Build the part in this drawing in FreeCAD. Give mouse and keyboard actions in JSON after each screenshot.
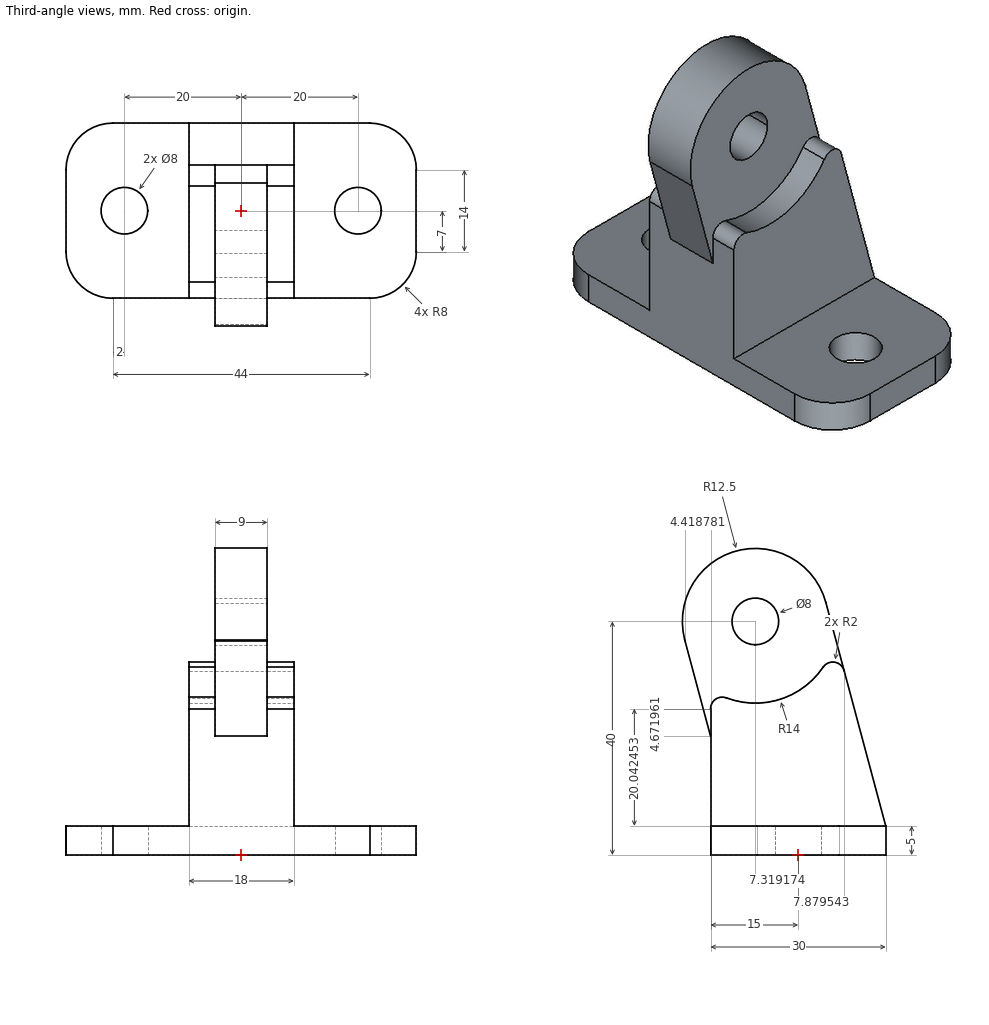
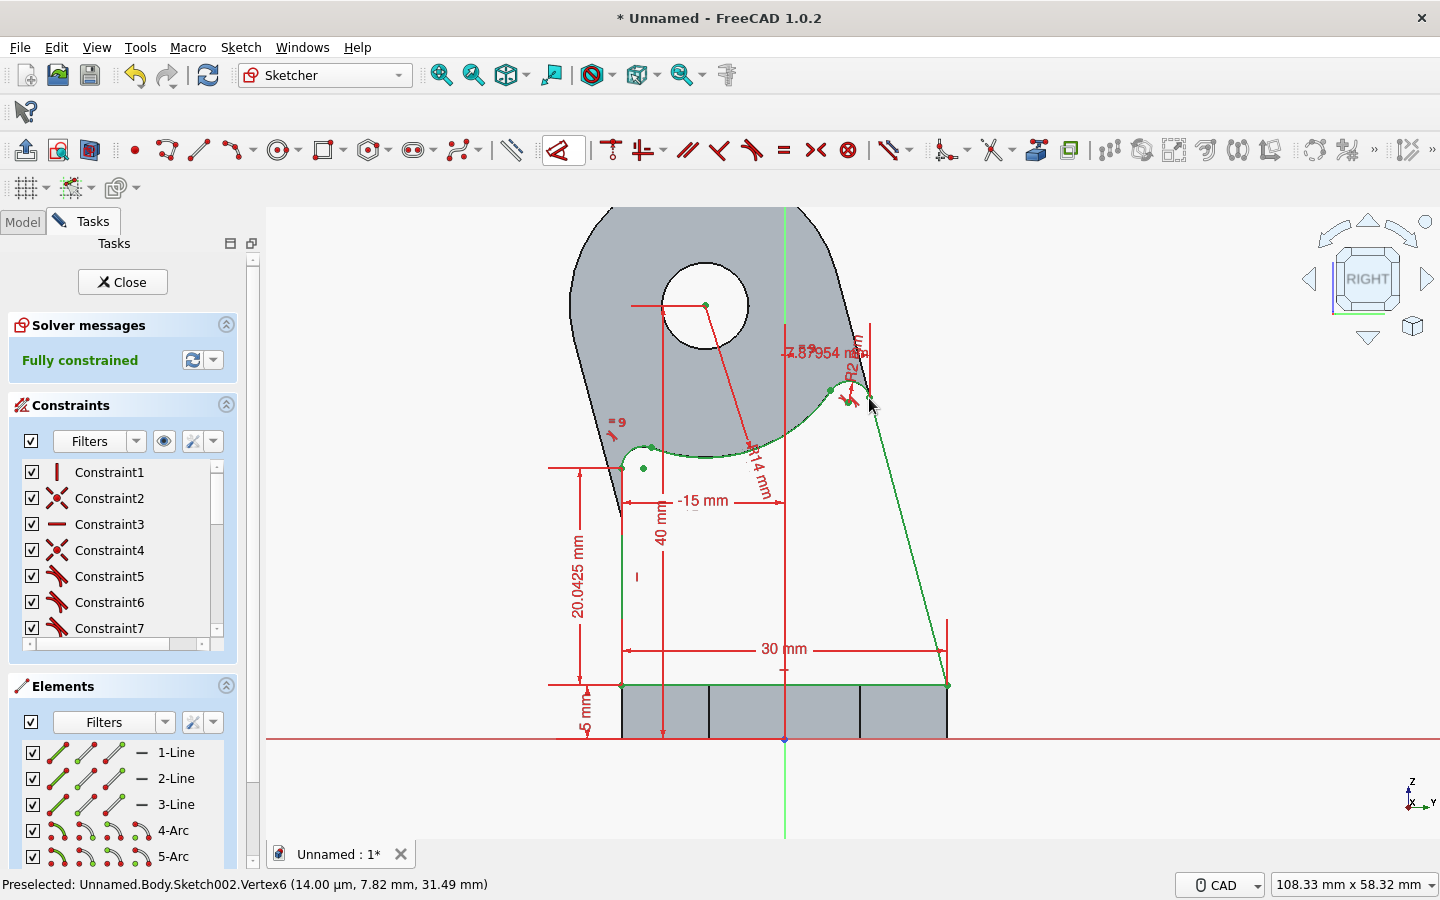
{"action": "left_click", "coordinate": [123, 282]}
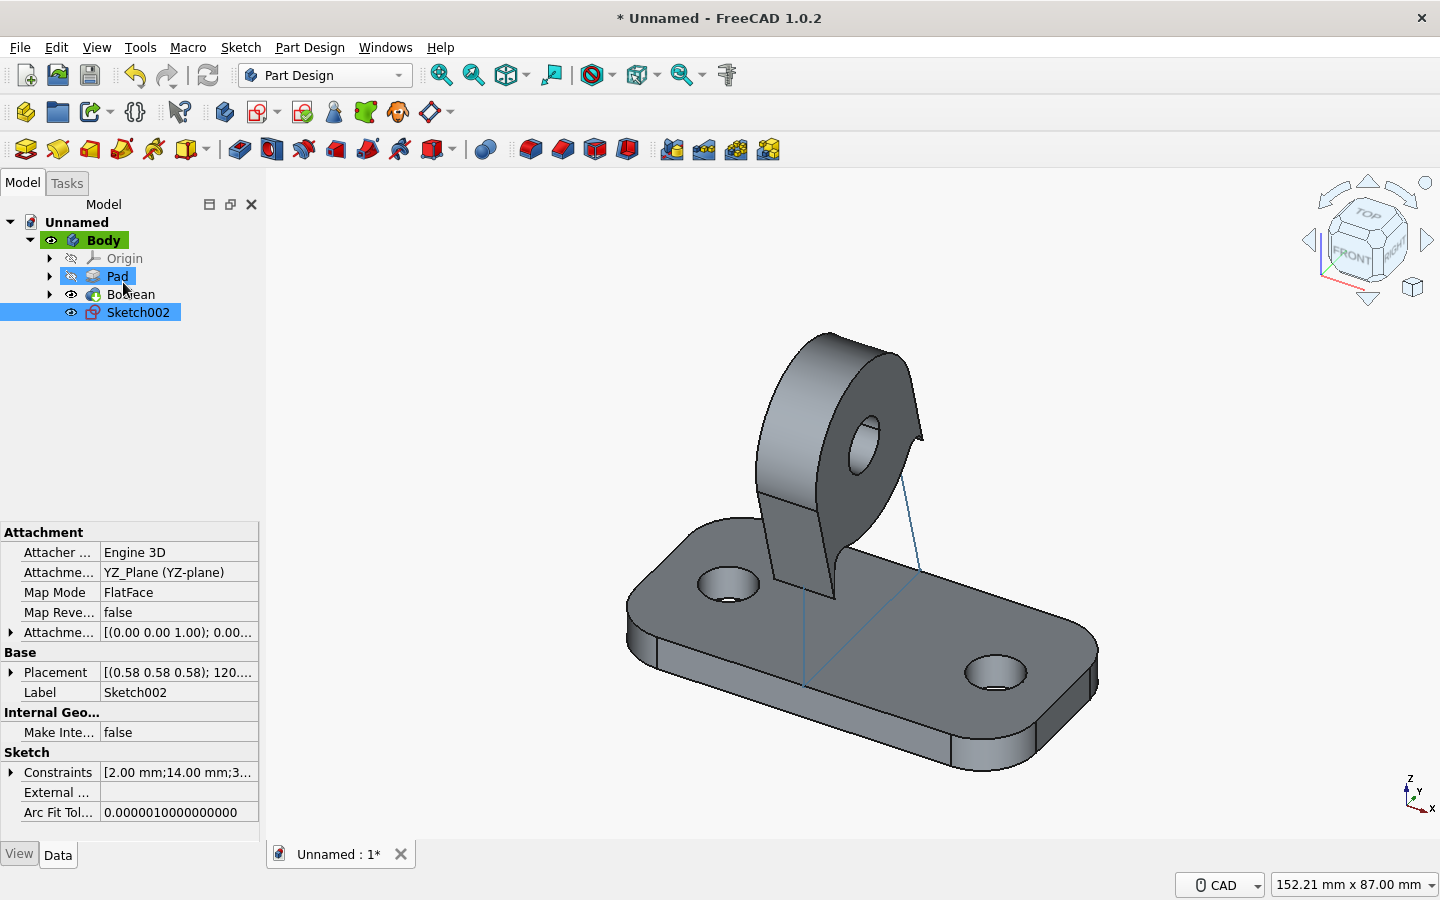
{"action": "left_click", "coordinate": [26, 150]}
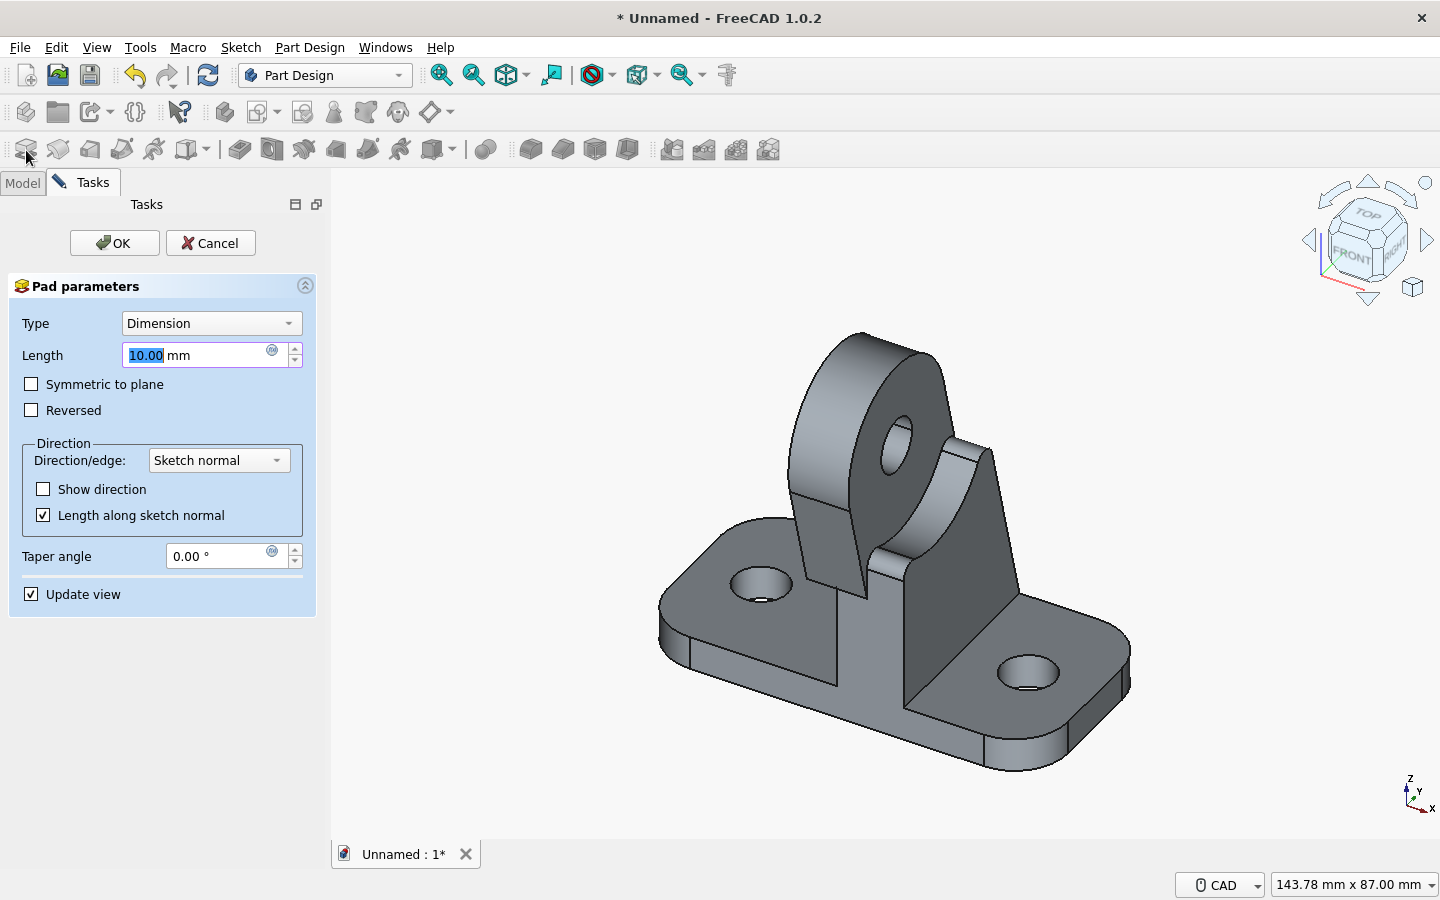
{"action": "type", "text": "18"}
{"action": "key", "text": "Tab"}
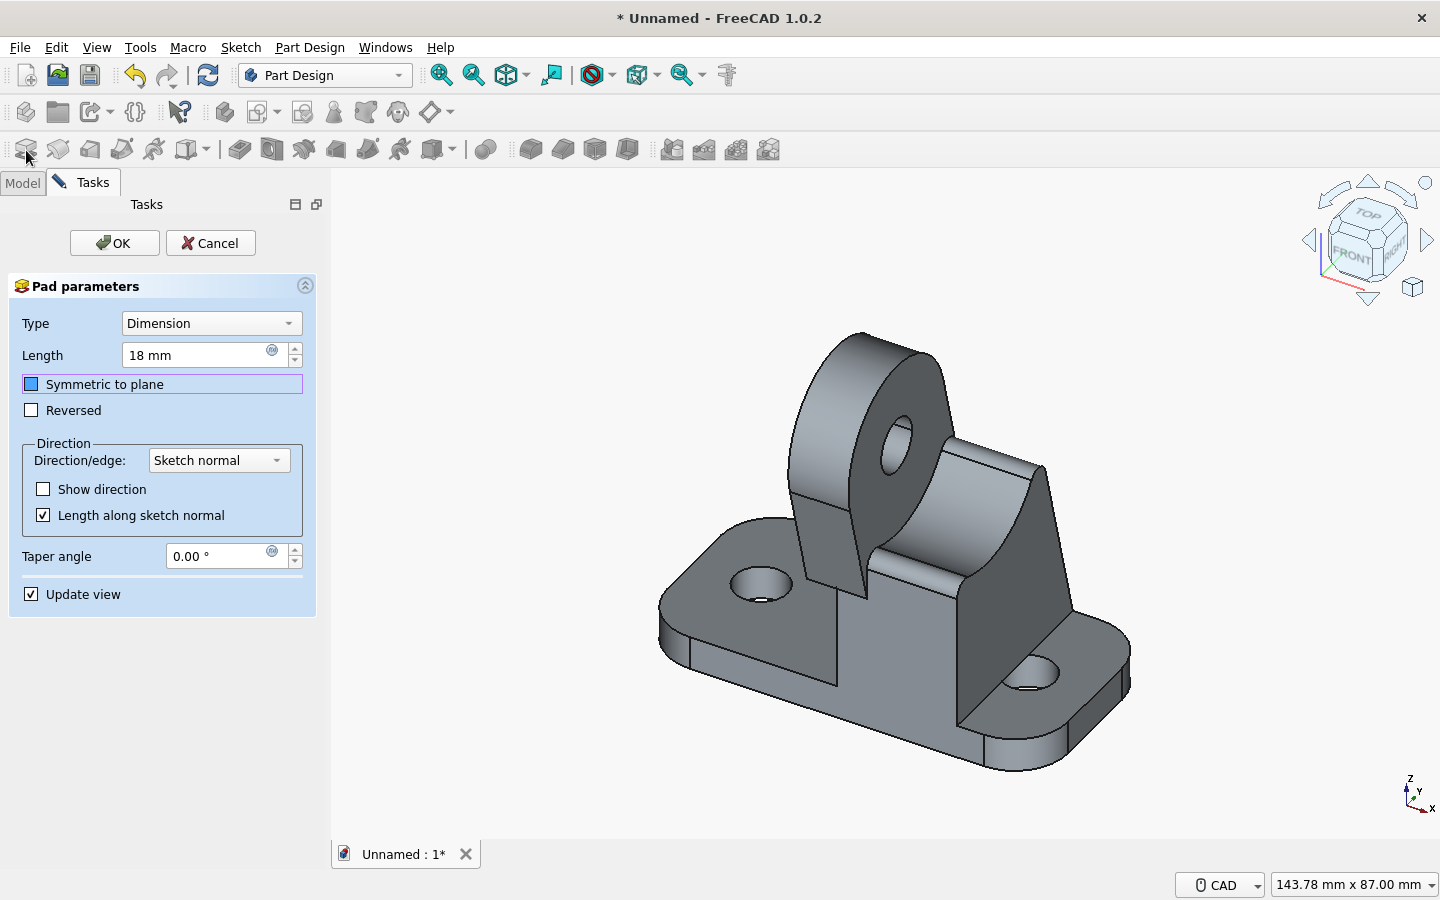
{"action": "left_click", "coordinate": [30, 384]}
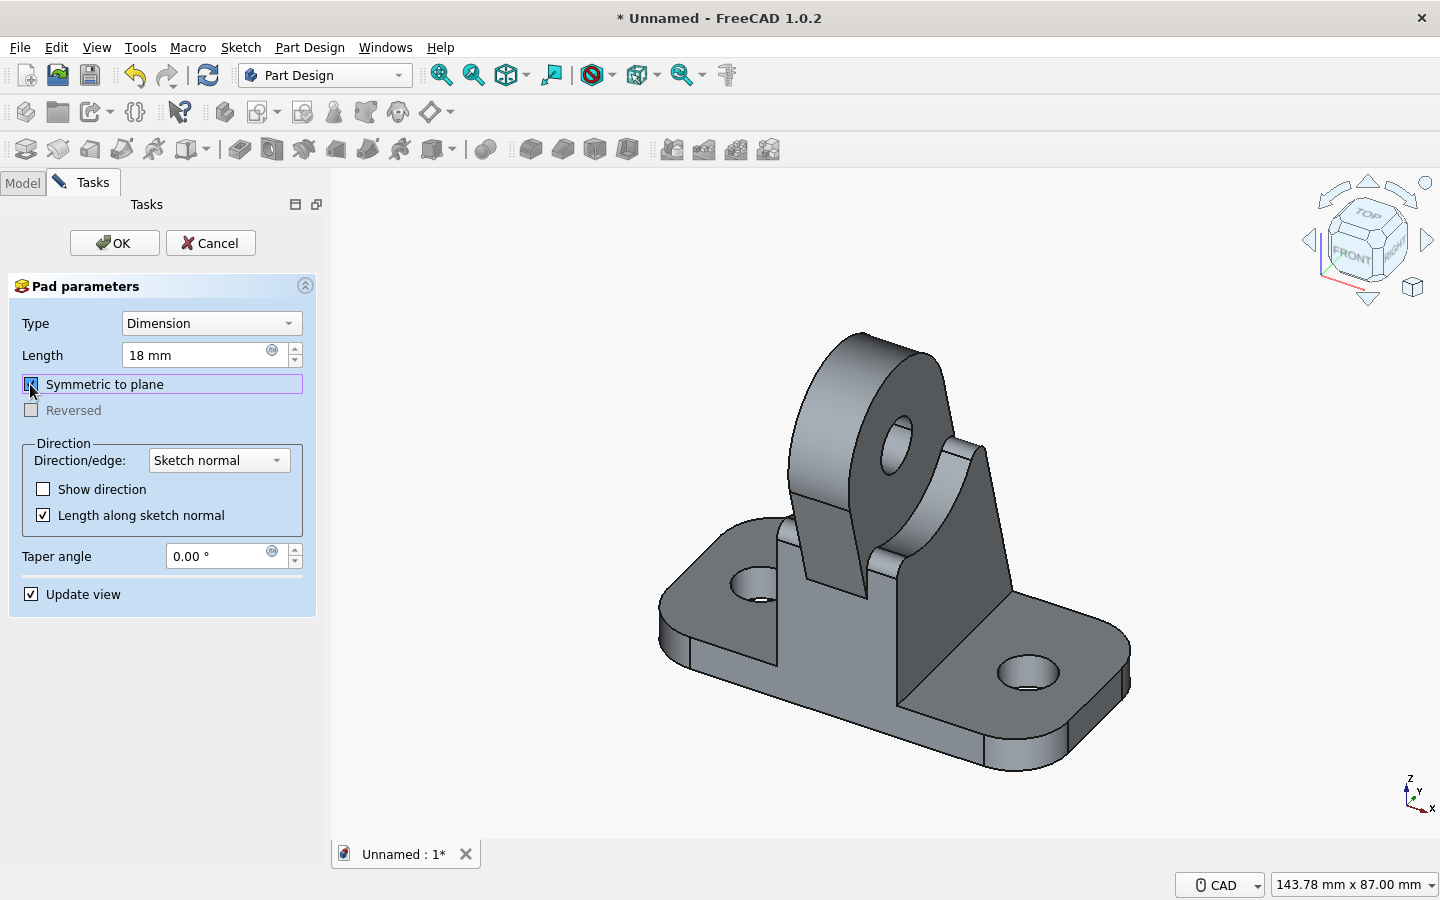
{"action": "left_click", "coordinate": [115, 243]}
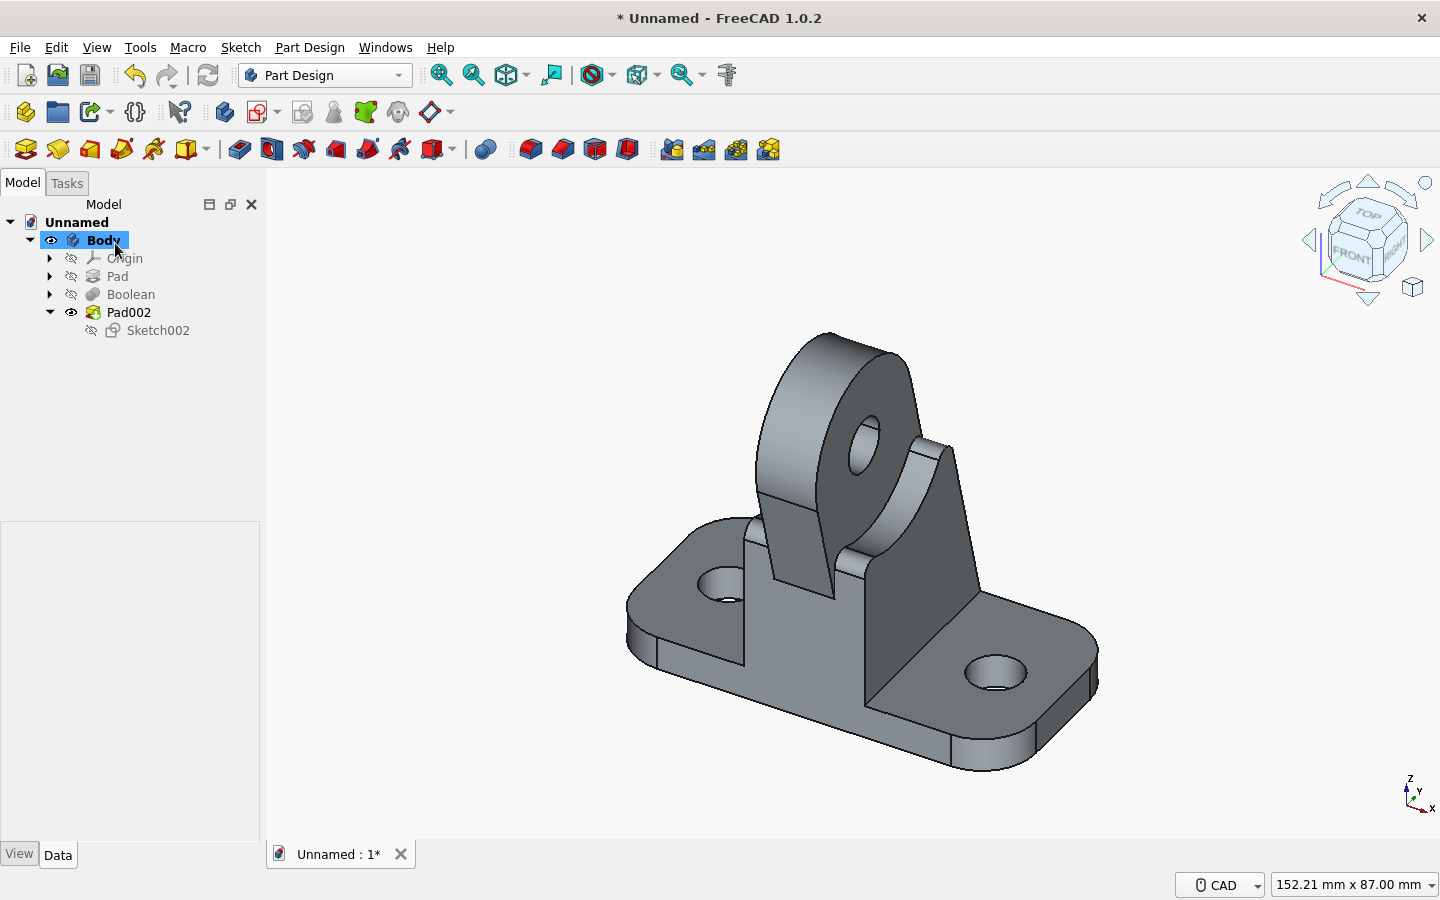
{"action": "key", "text": "0"}